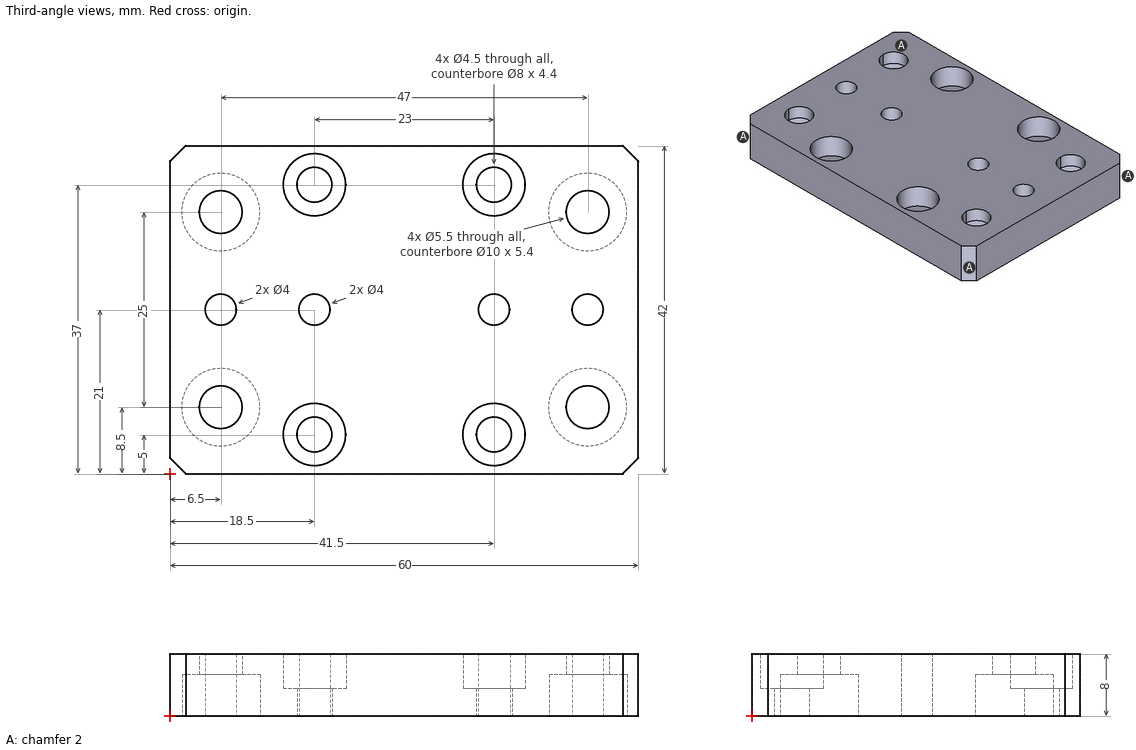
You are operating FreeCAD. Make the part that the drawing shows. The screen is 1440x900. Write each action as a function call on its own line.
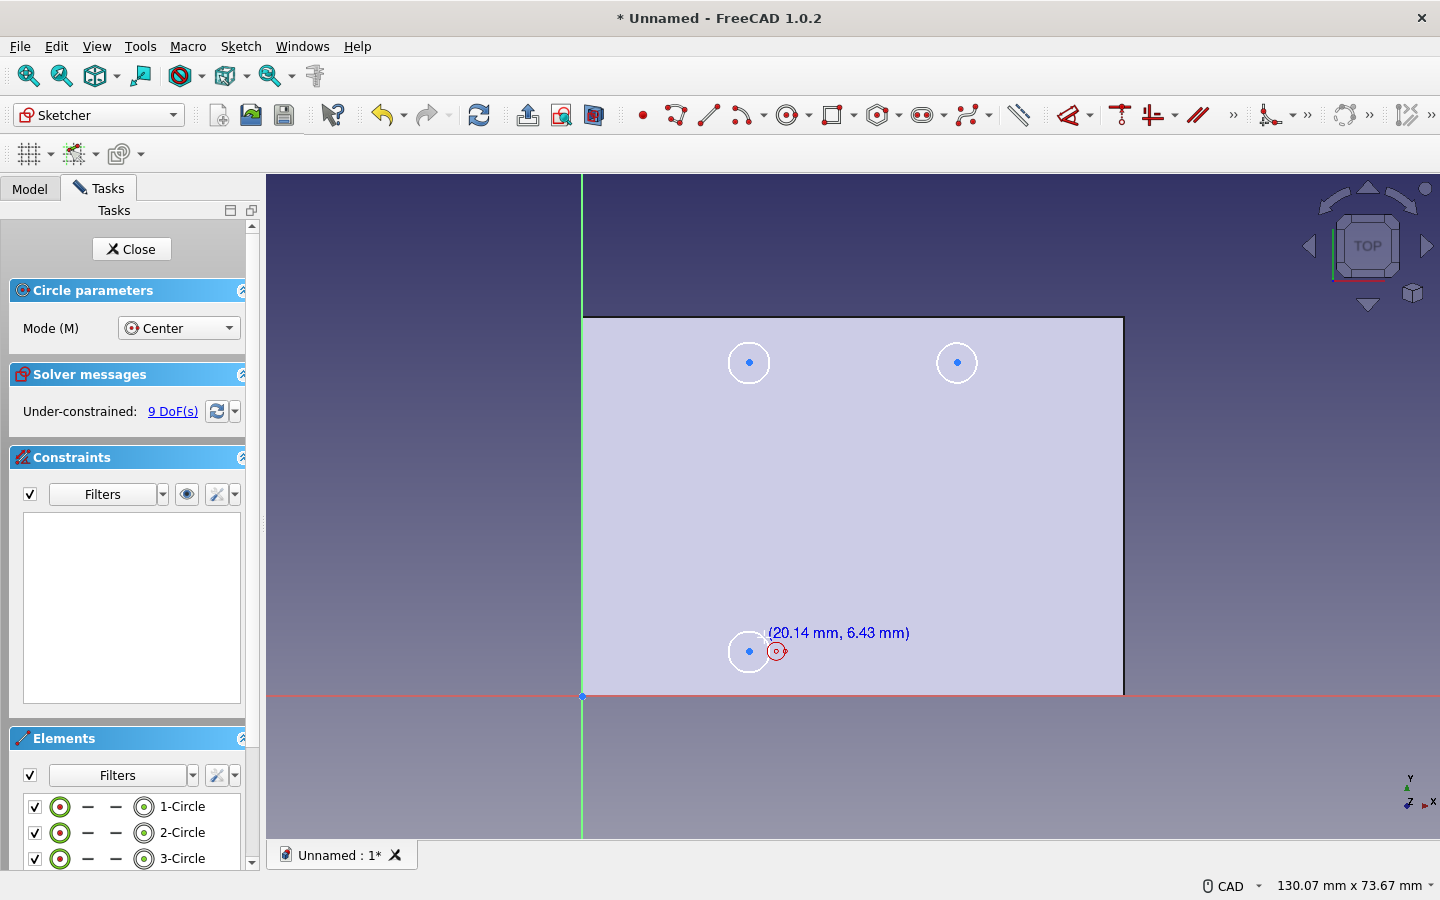
click(957, 651)
click(971, 637)
key(Escape)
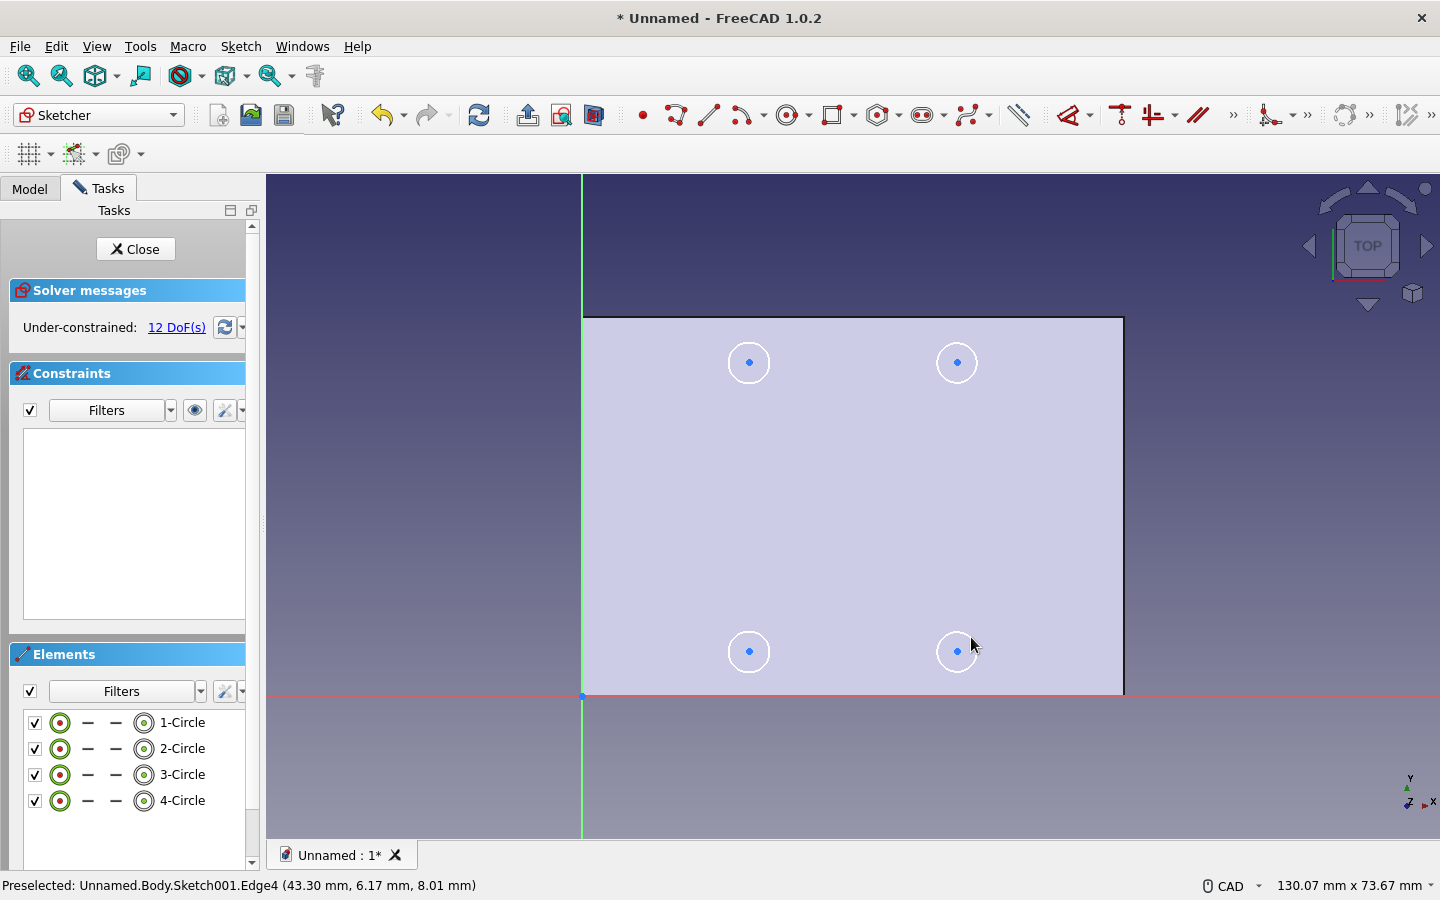
click(971, 349)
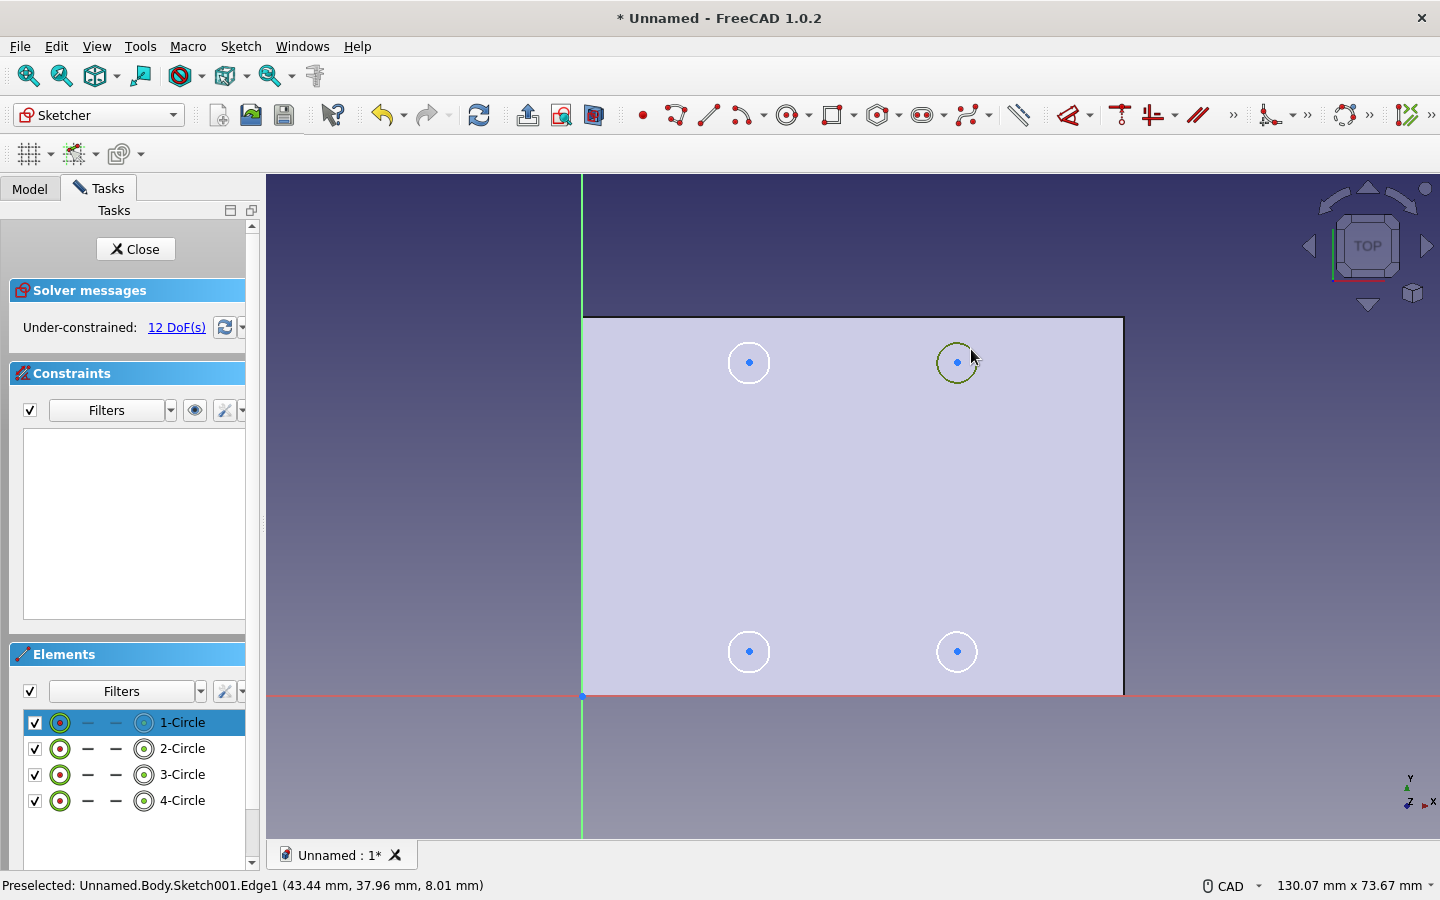
click(763, 348)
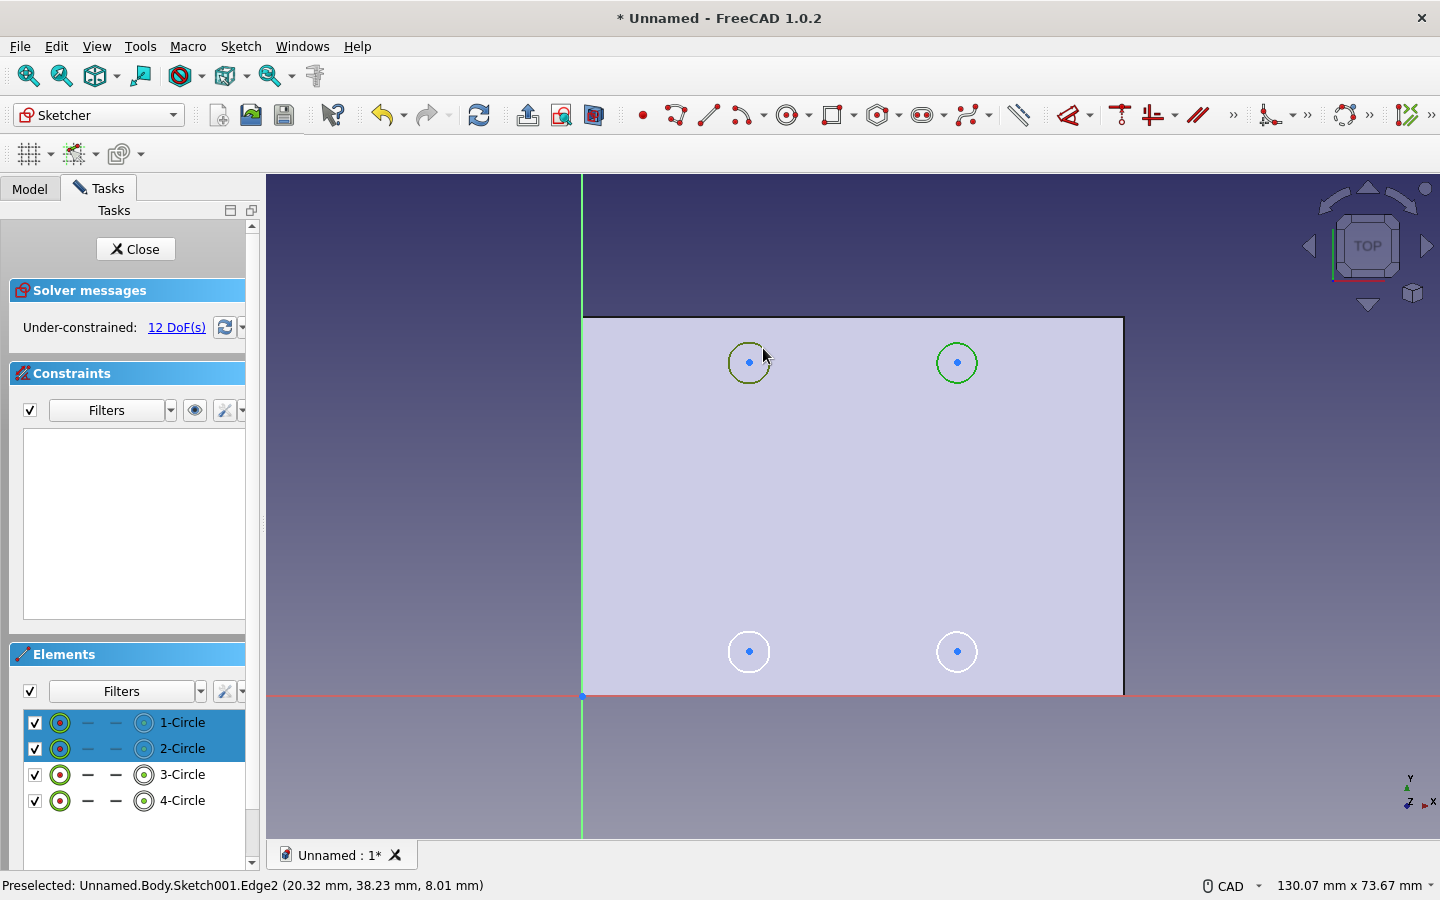
click(763, 637)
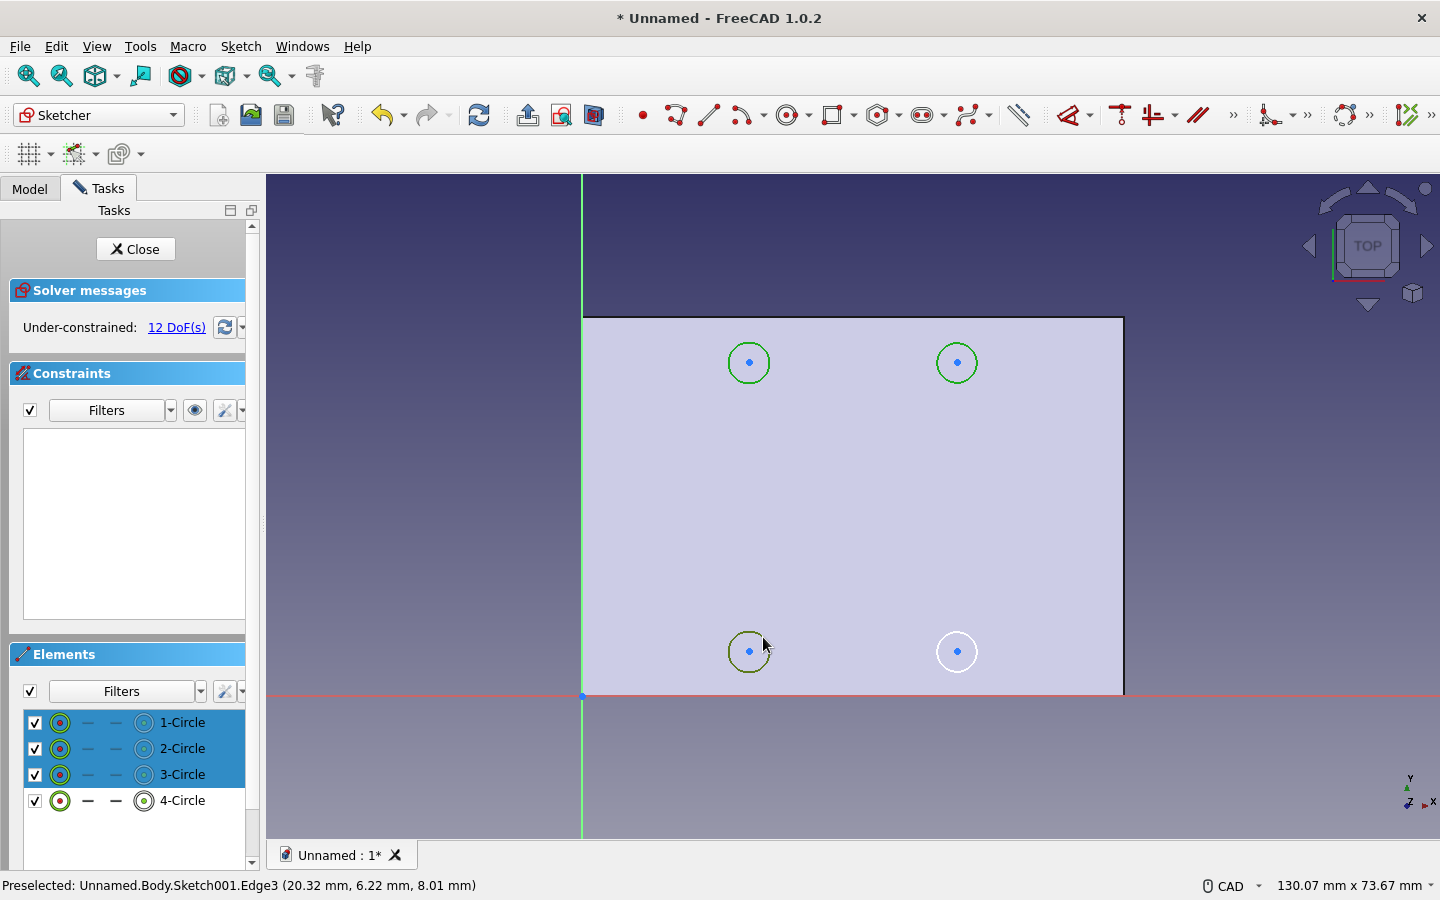
click(971, 638)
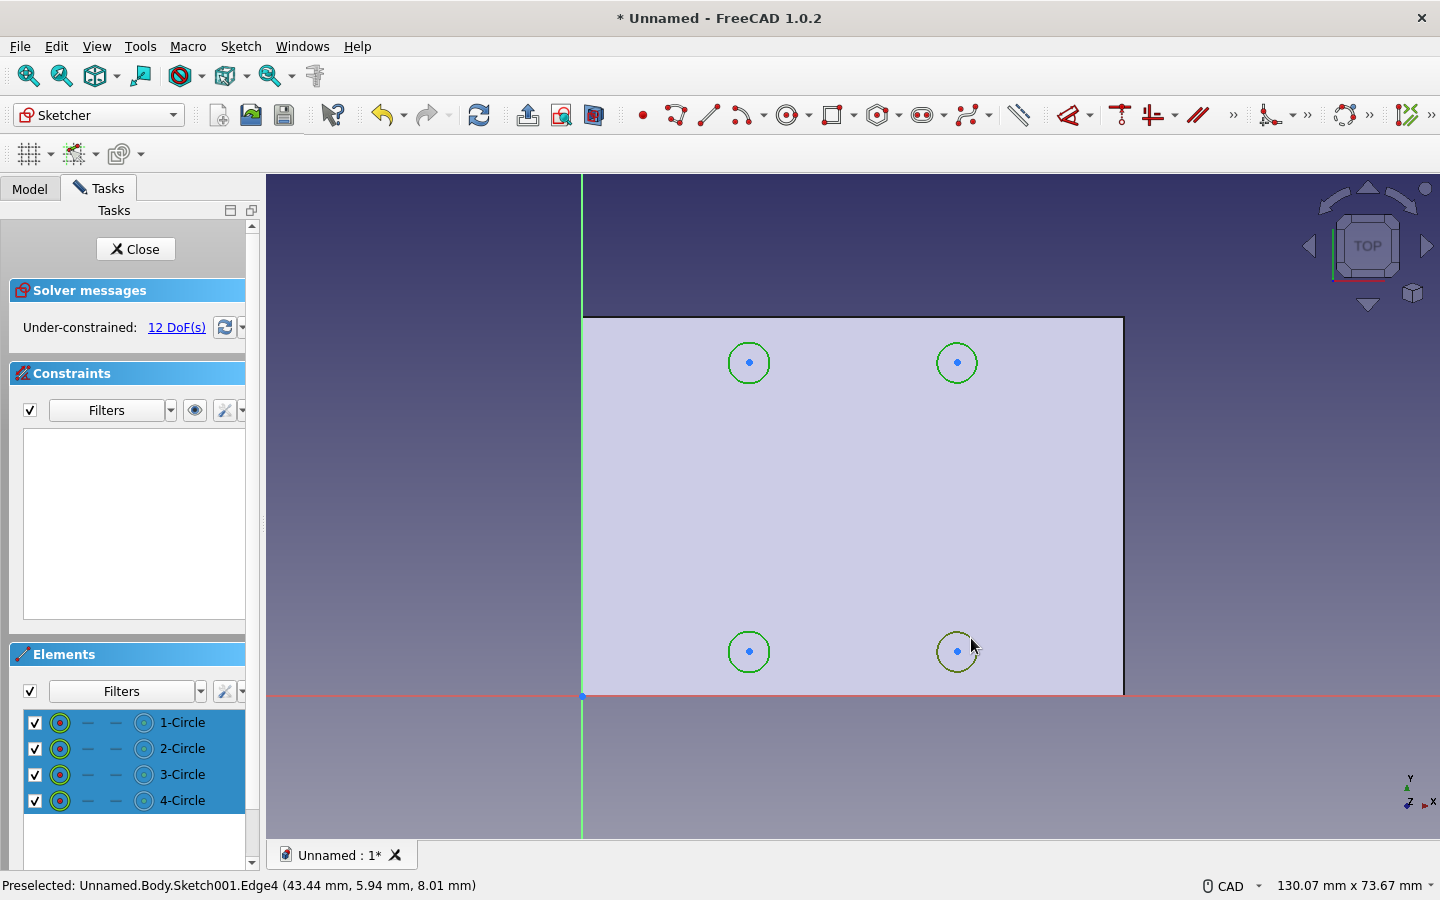
key(e)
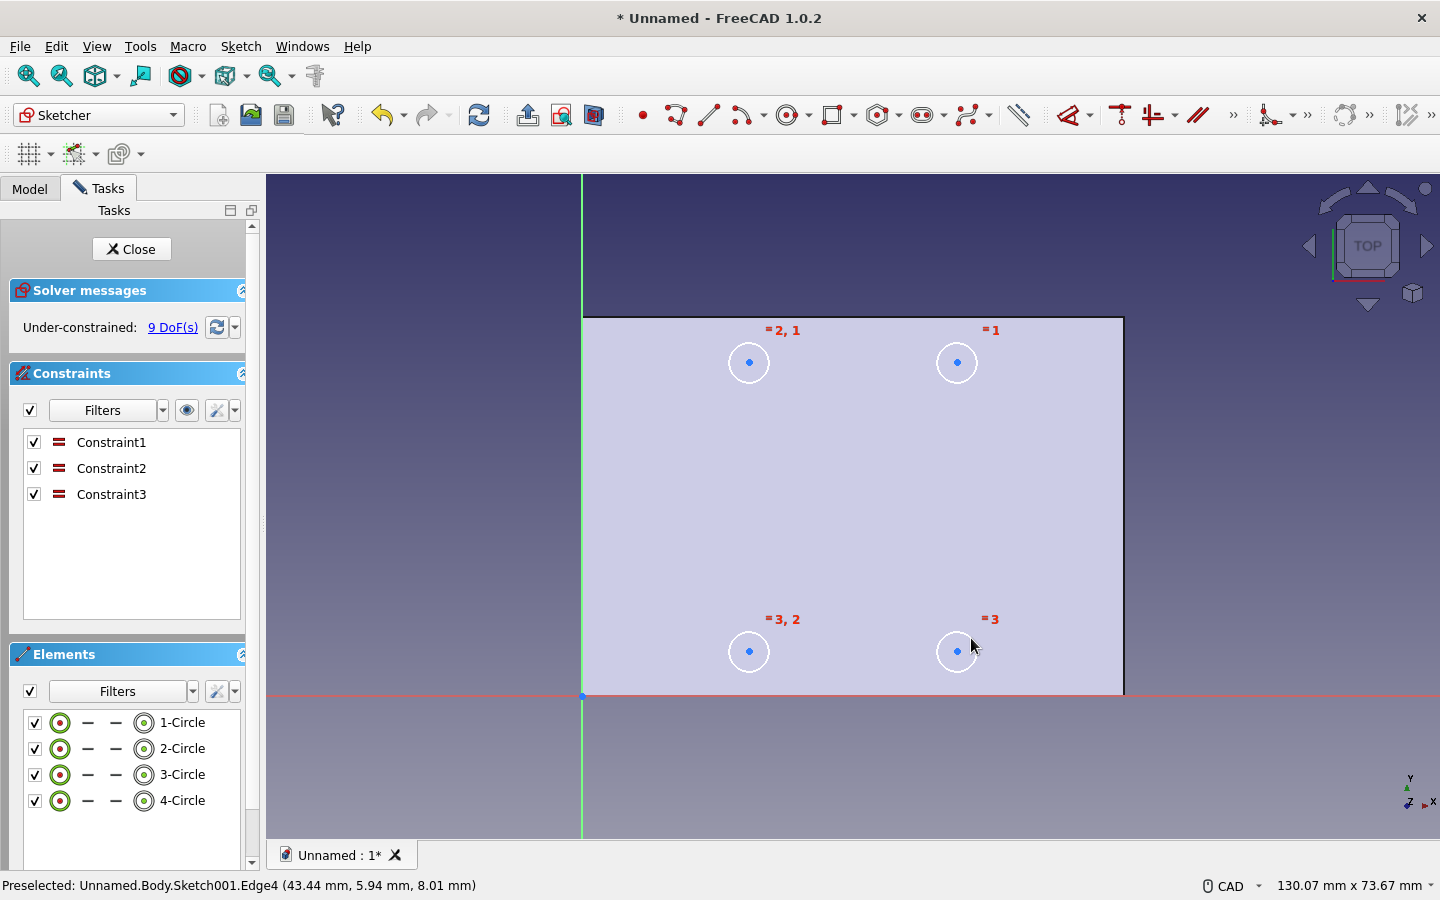
click(957, 363)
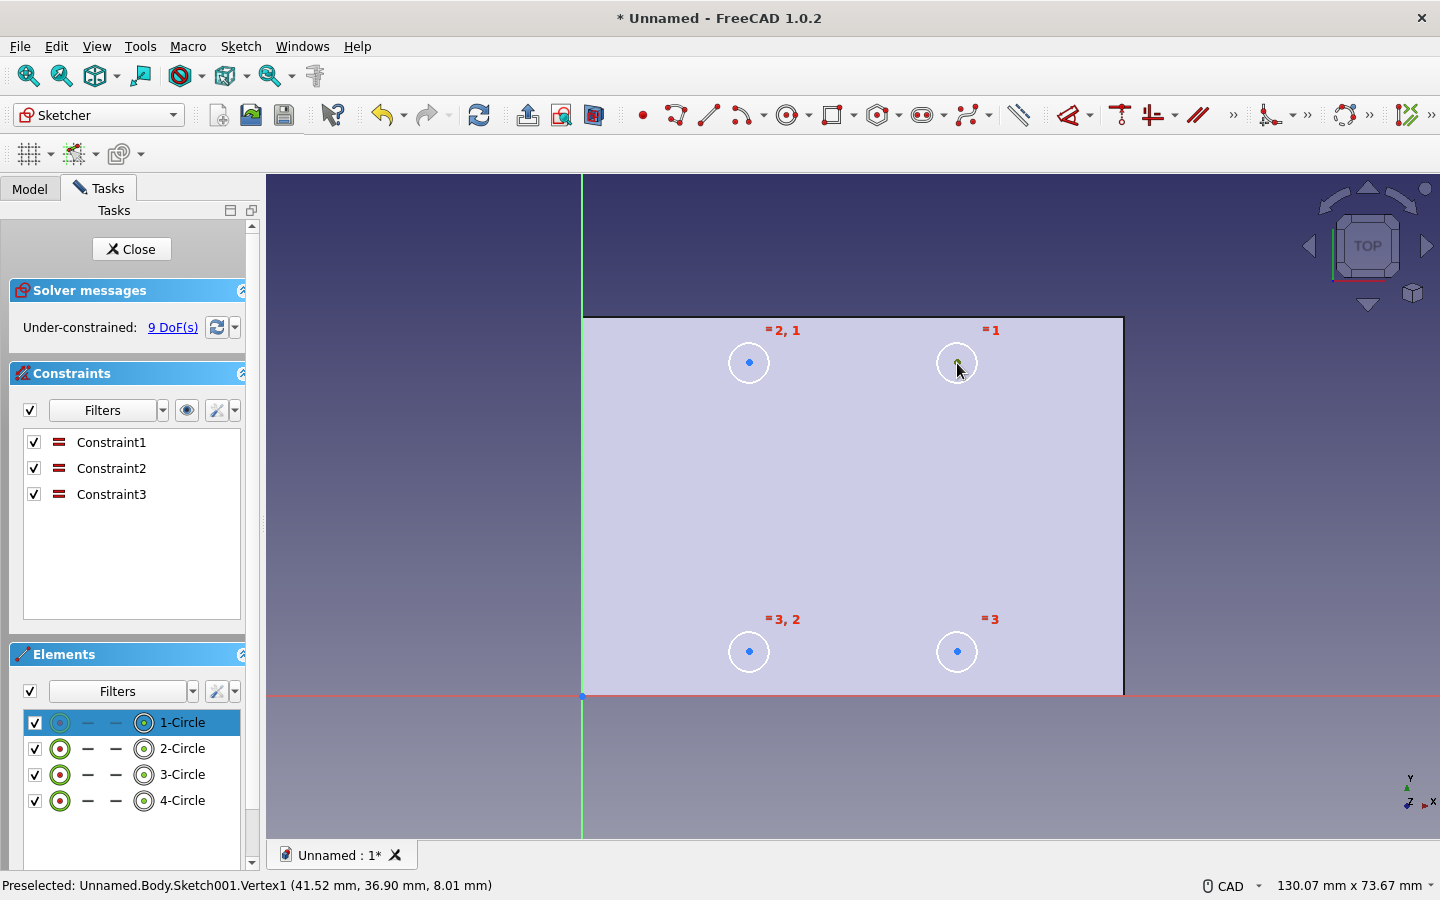
click(749, 363)